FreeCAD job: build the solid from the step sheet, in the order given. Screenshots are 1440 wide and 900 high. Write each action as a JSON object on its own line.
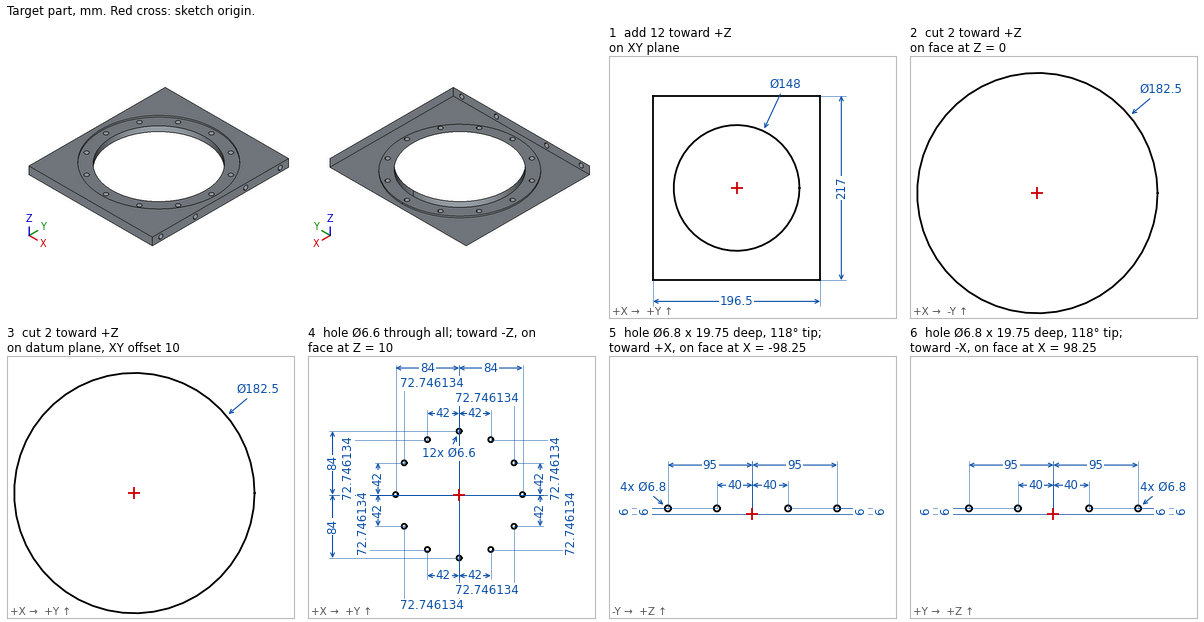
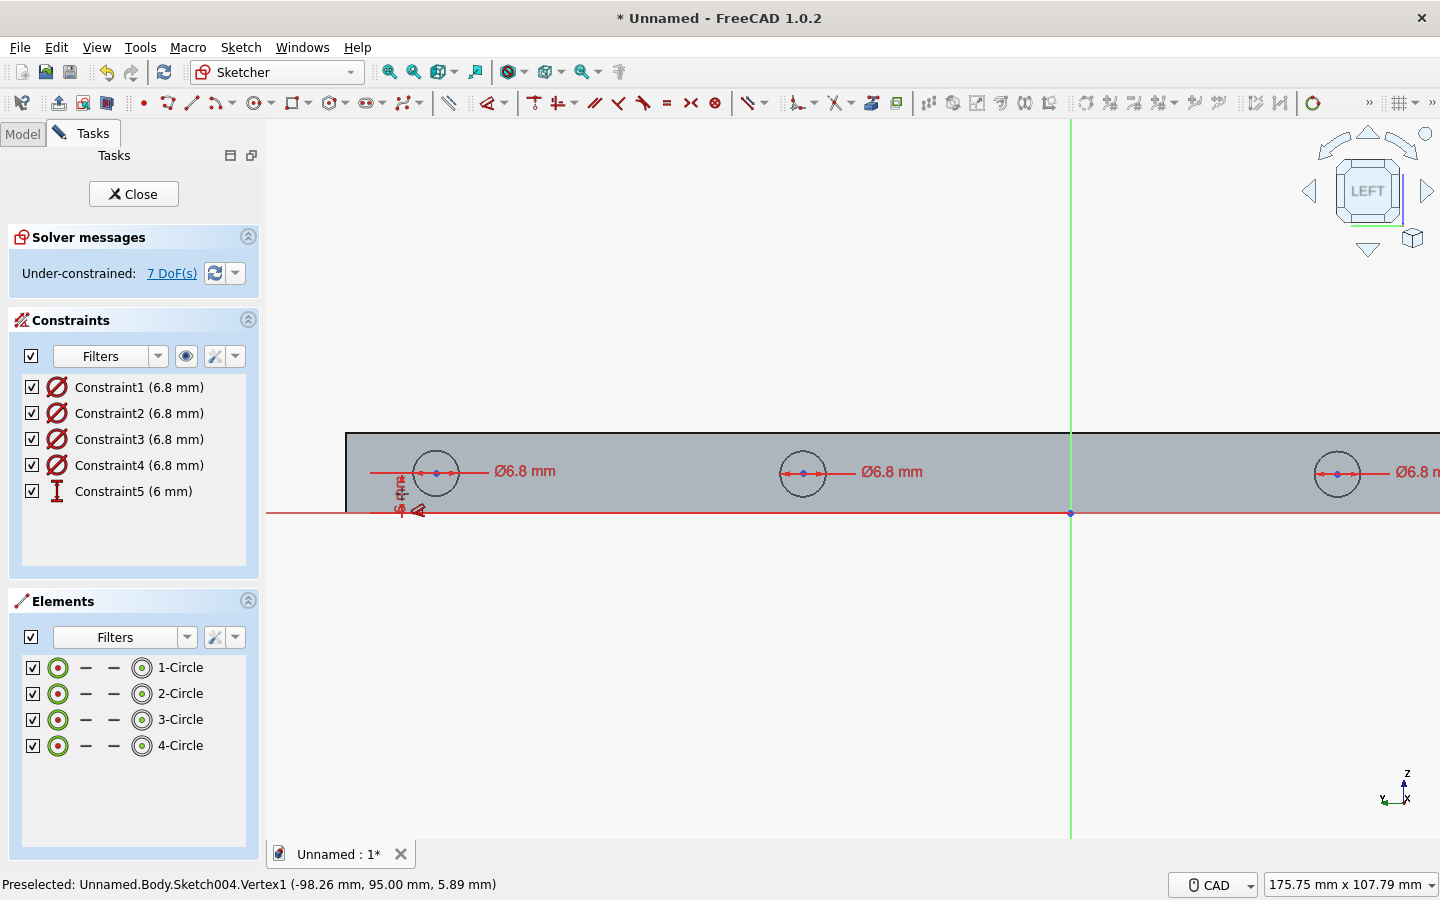
{"action": "left_click", "coordinate": [803, 474]}
{"action": "left_click", "coordinate": [769, 494]}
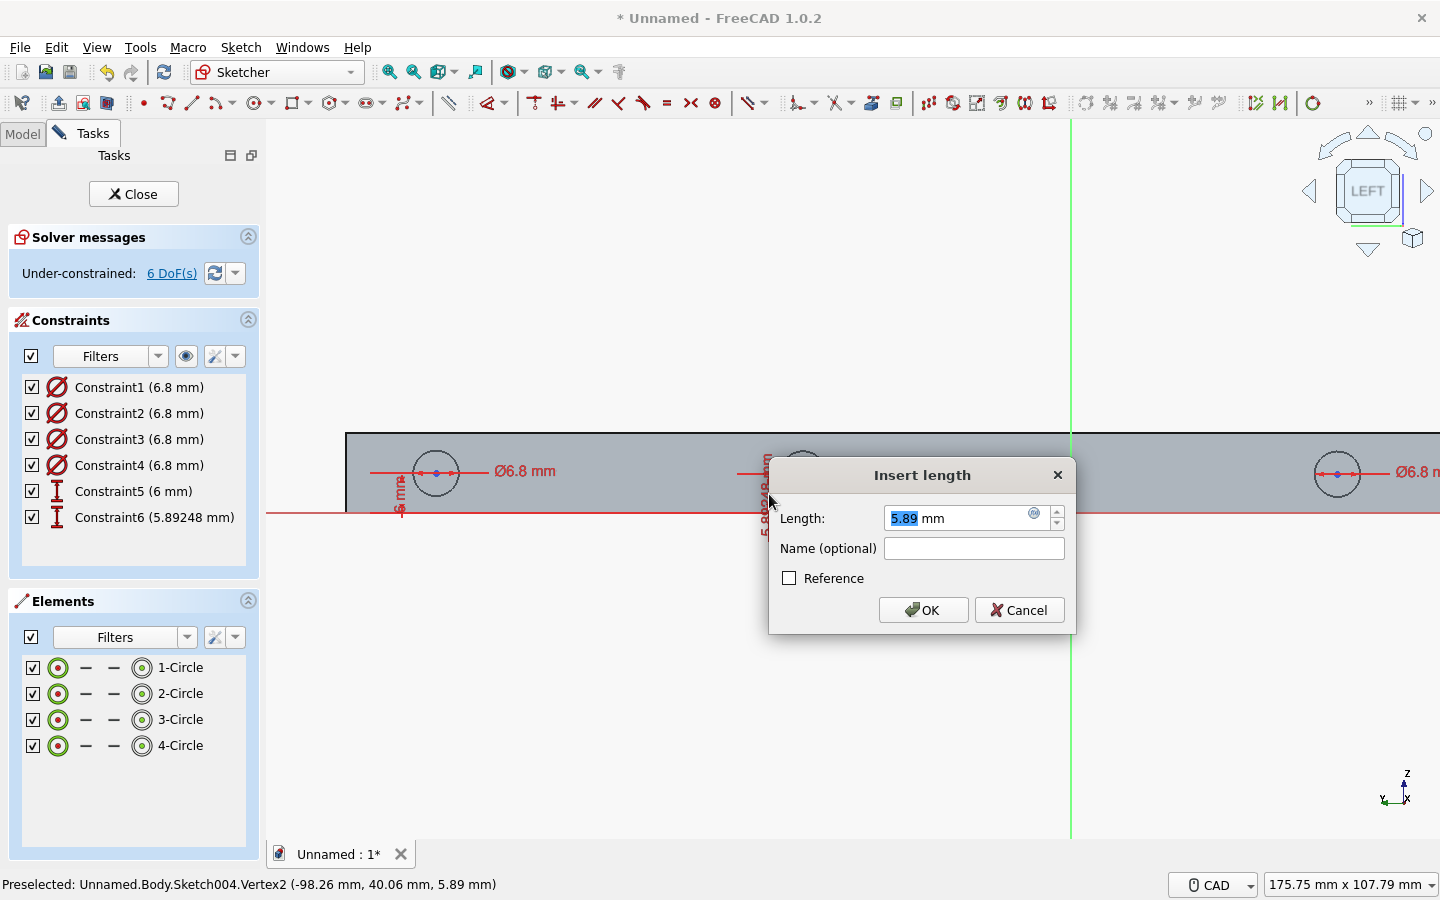
{"action": "type", "text": "6"}
{"action": "key", "text": "Return"}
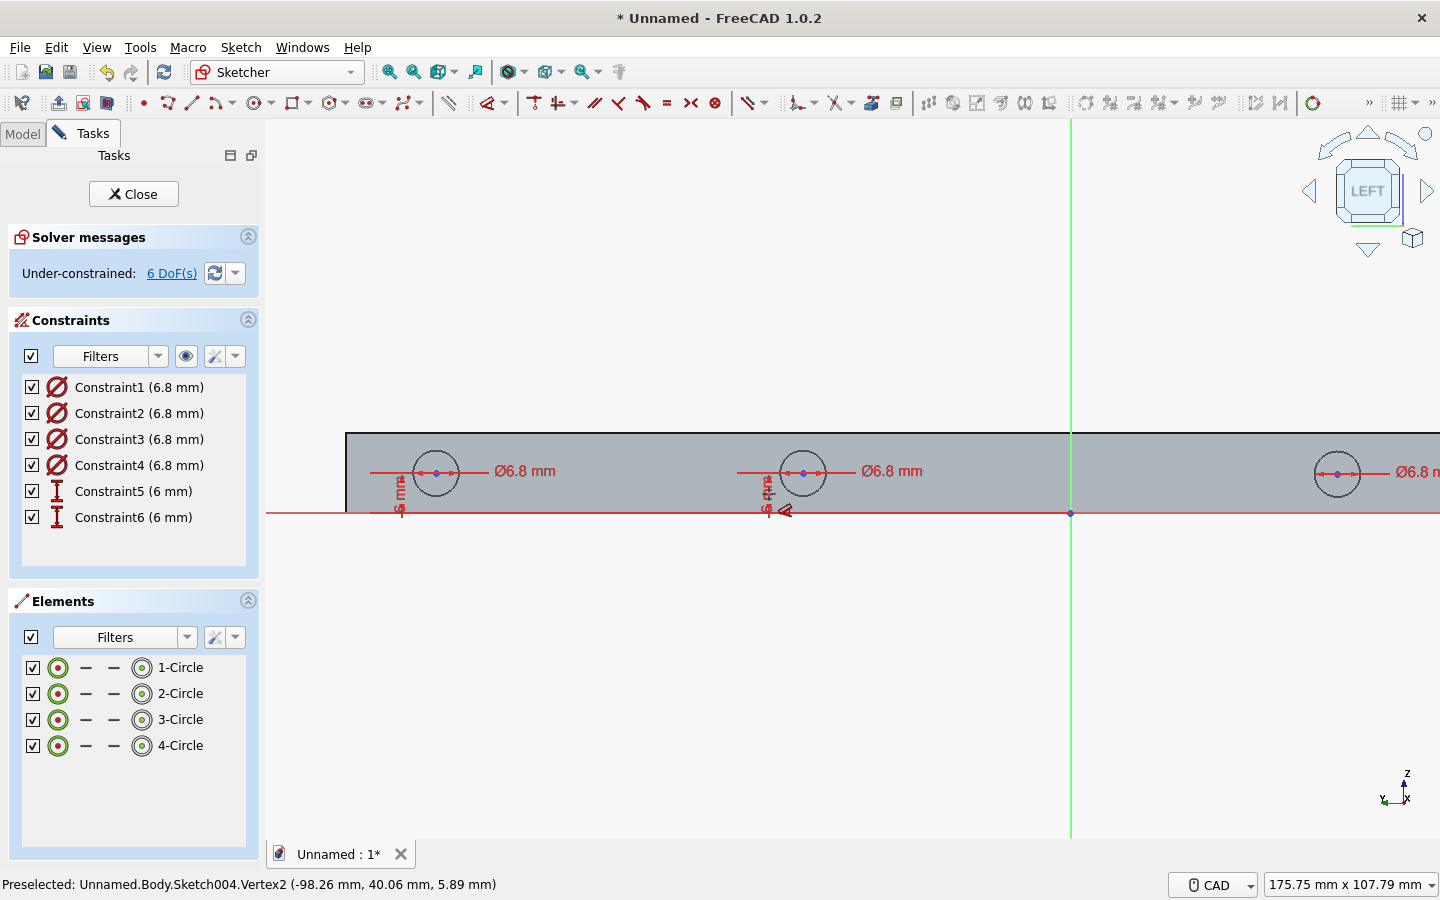
{"action": "scroll", "coordinate": [437, 475], "scroll_direction": "down", "scroll_amount": 3}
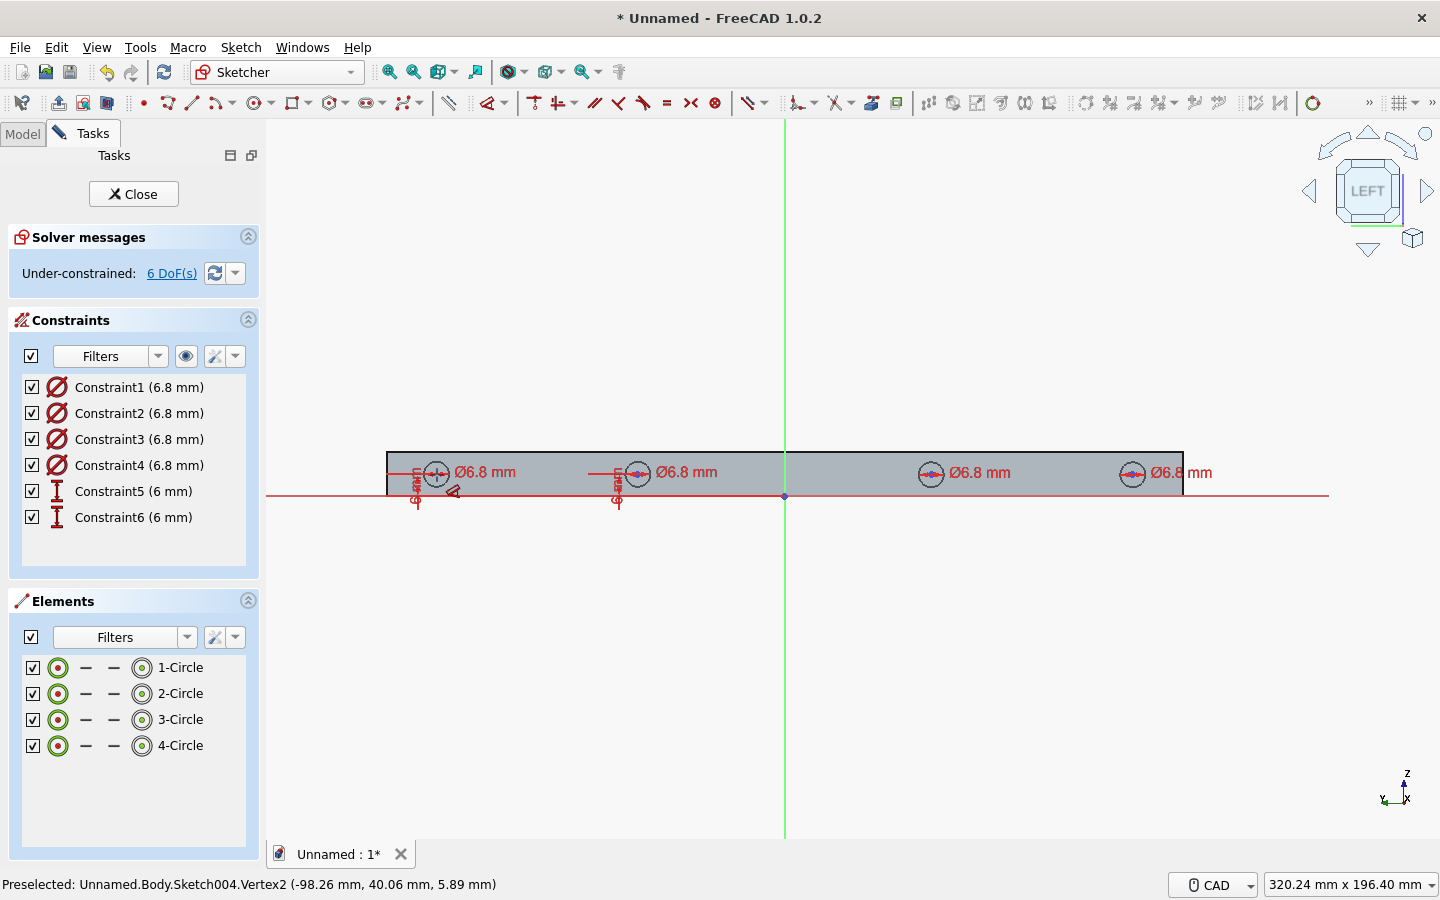
{"action": "scroll", "coordinate": [931, 475], "scroll_direction": "up", "scroll_amount": 3}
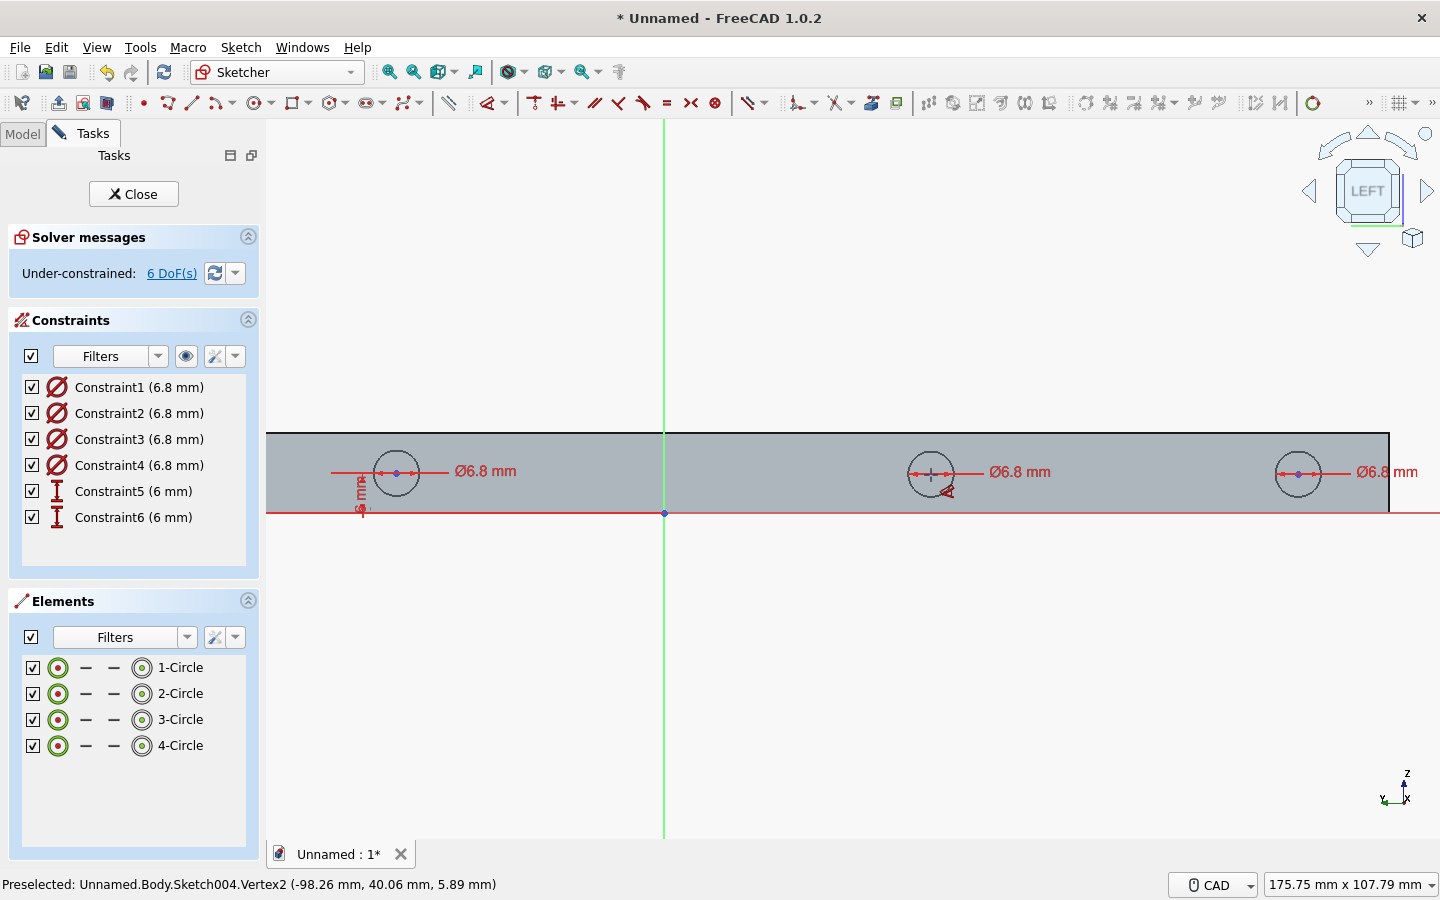
{"action": "left_click", "coordinate": [931, 474]}
{"action": "left_click", "coordinate": [965, 494]}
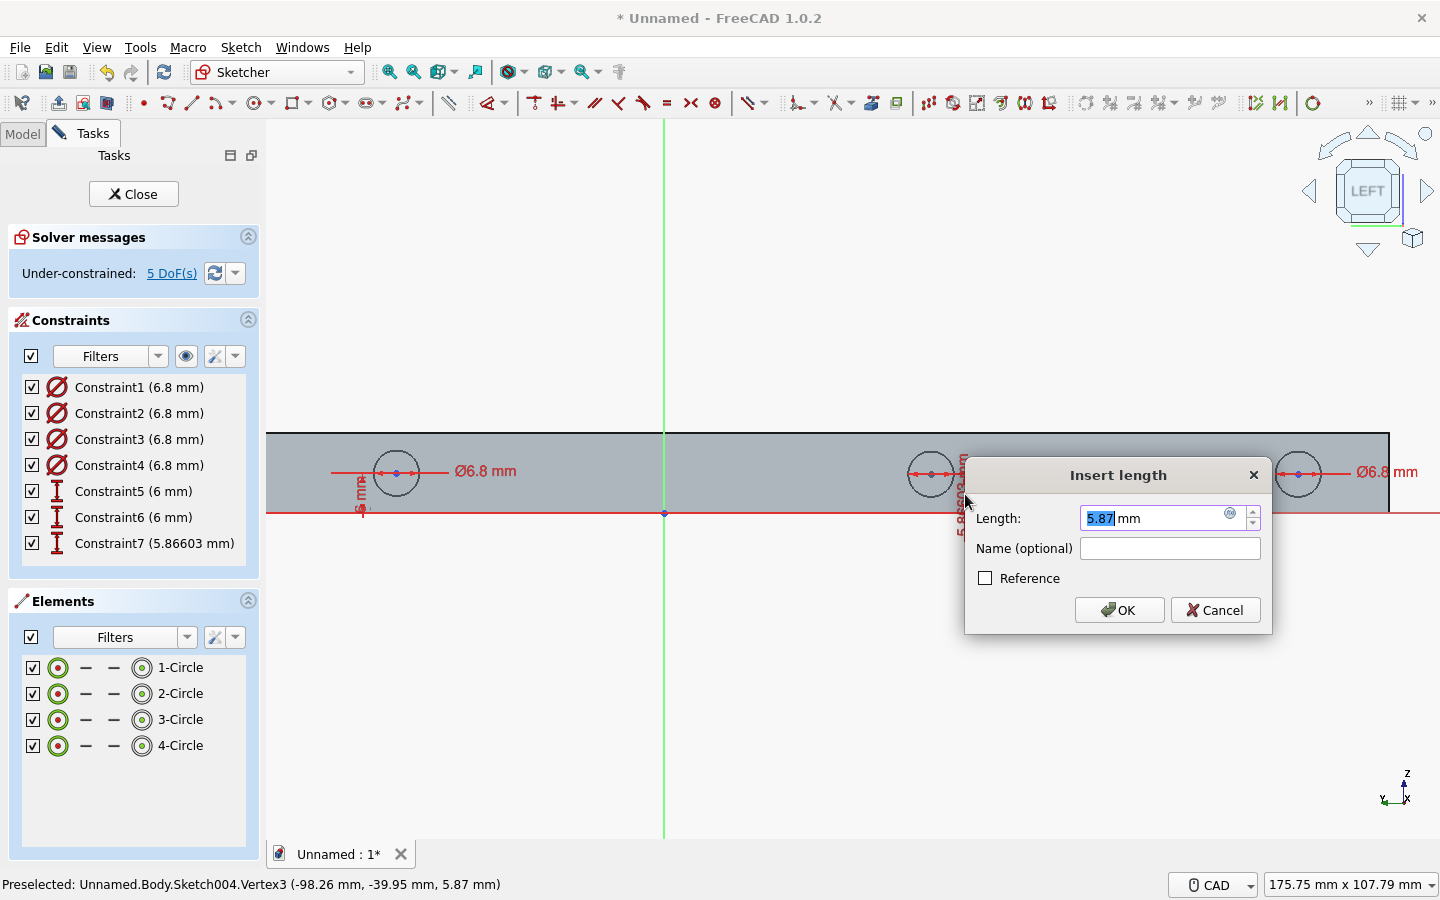
{"action": "type", "text": "6"}
{"action": "key", "text": "Return"}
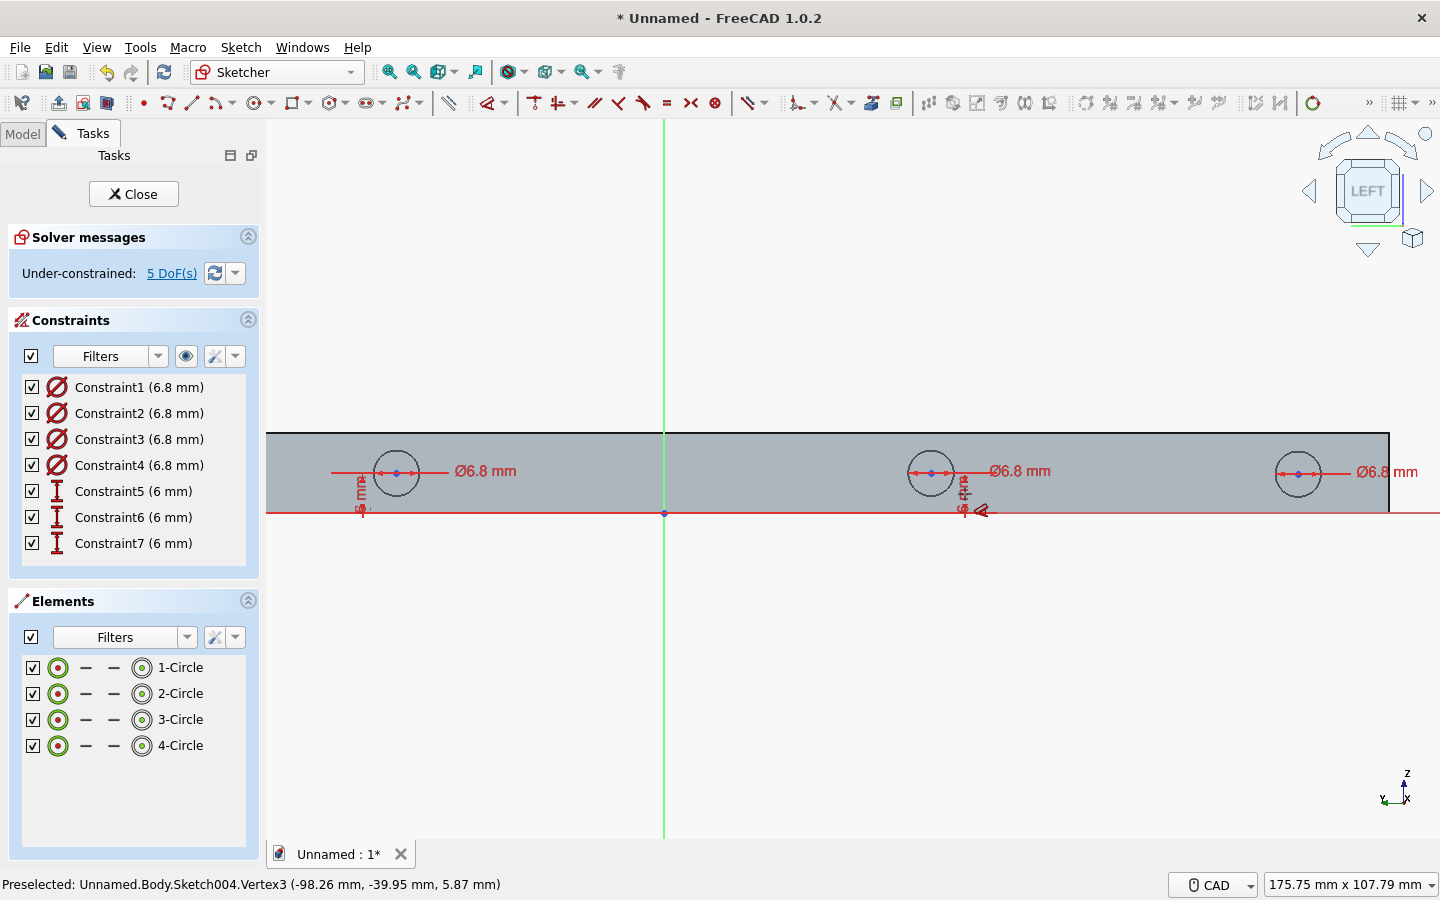
{"action": "scroll", "coordinate": [931, 475], "scroll_direction": "down", "scroll_amount": 3}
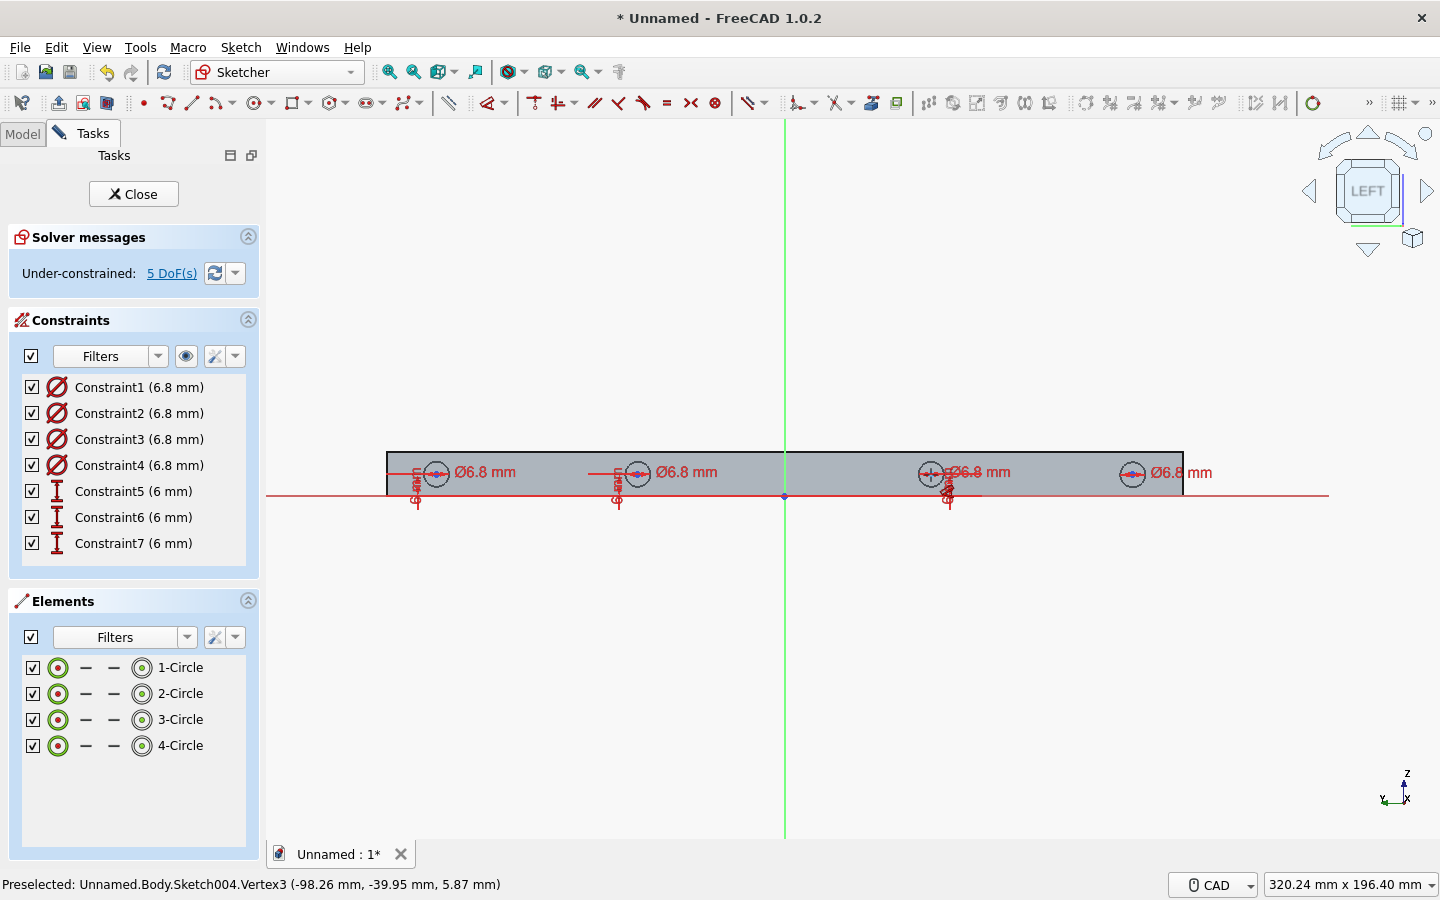
{"action": "scroll", "coordinate": [1133, 475], "scroll_direction": "up", "scroll_amount": 3}